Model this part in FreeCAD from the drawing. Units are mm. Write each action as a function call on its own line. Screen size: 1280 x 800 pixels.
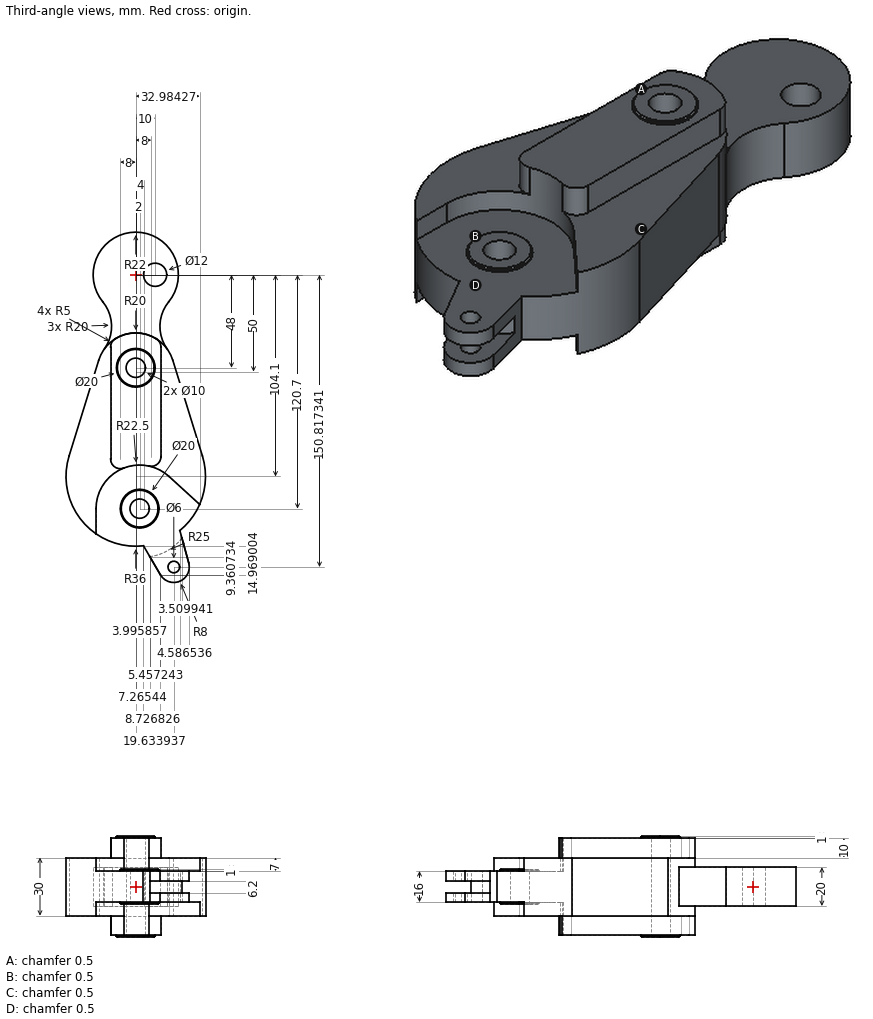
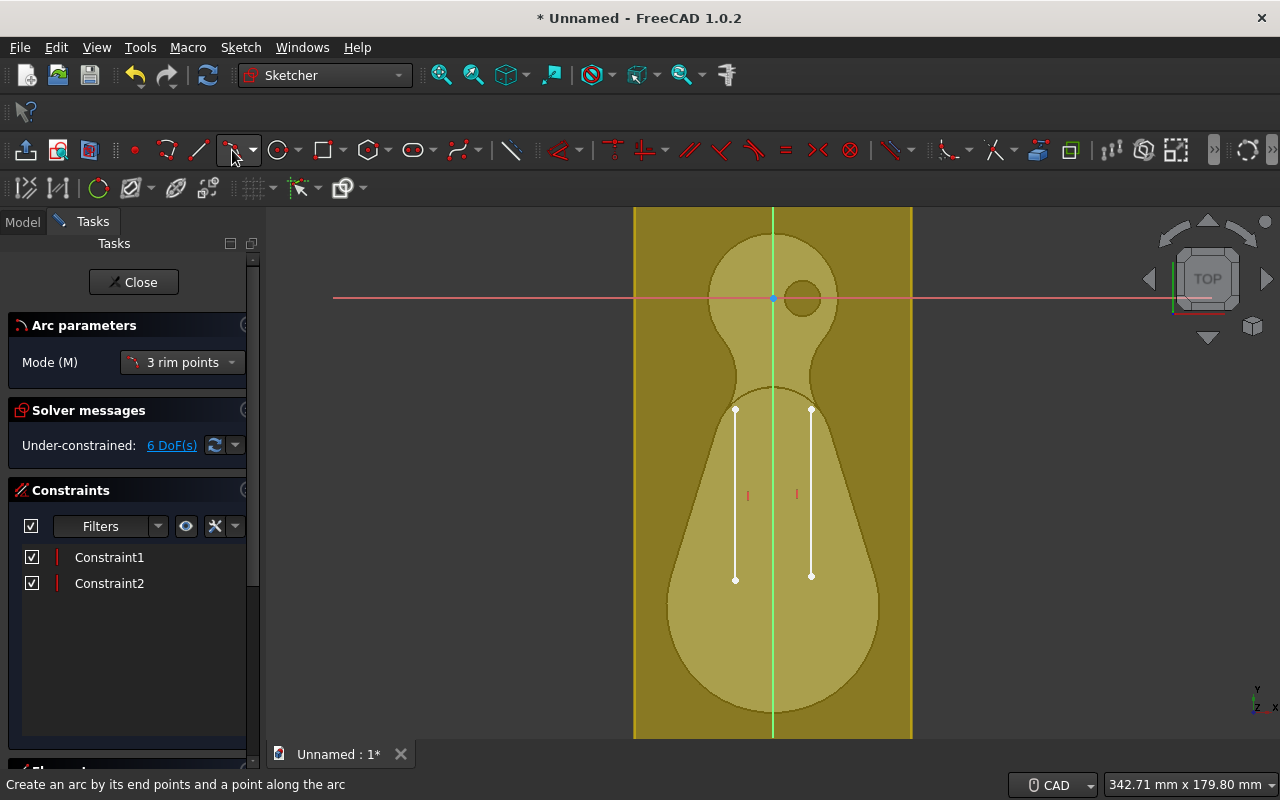
click(735, 581)
click(755, 594)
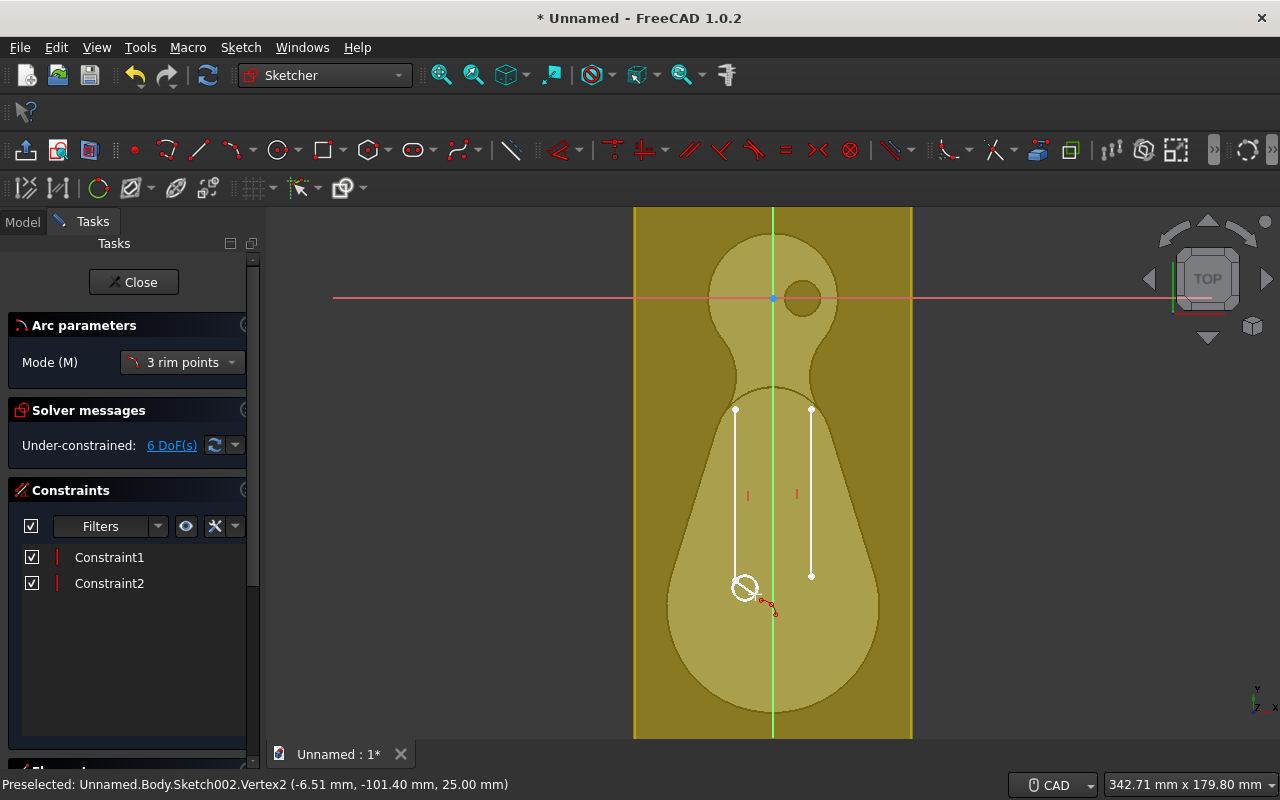
scroll(741, 592, up, 5)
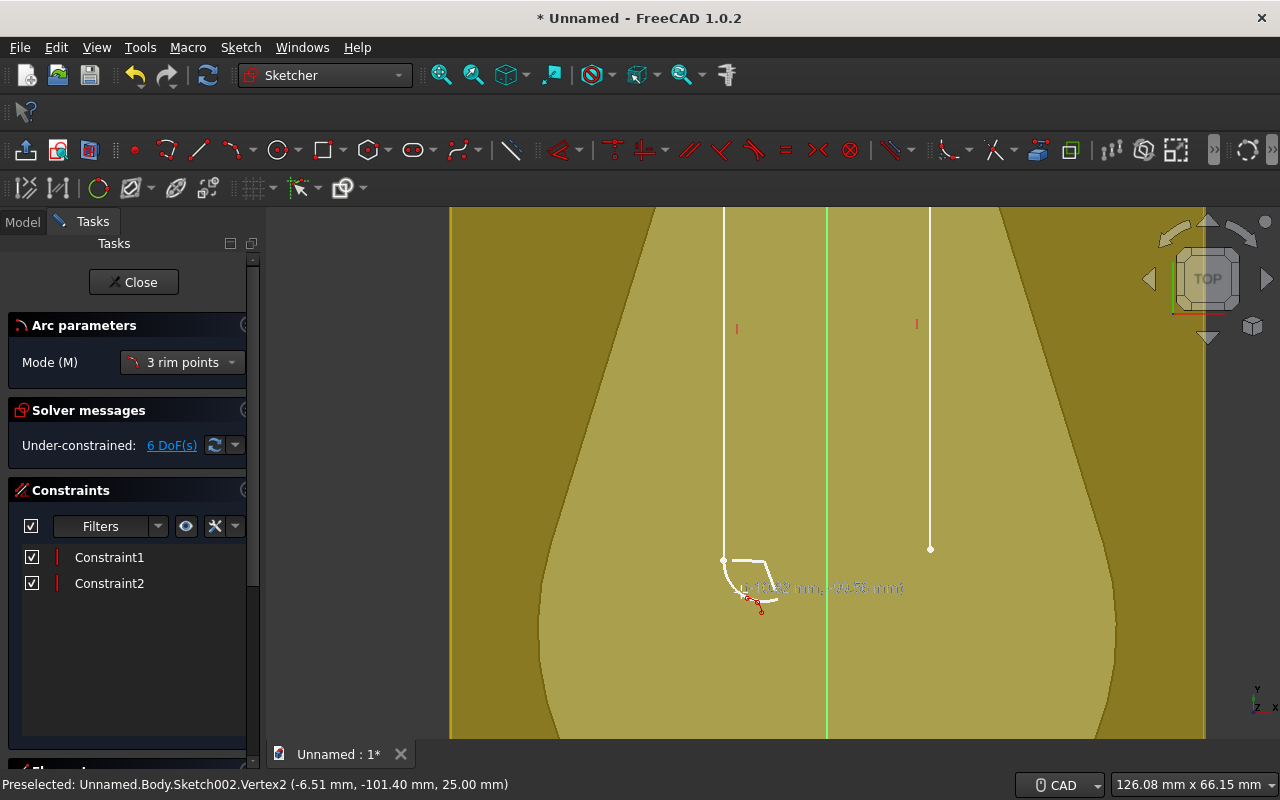
click(740, 591)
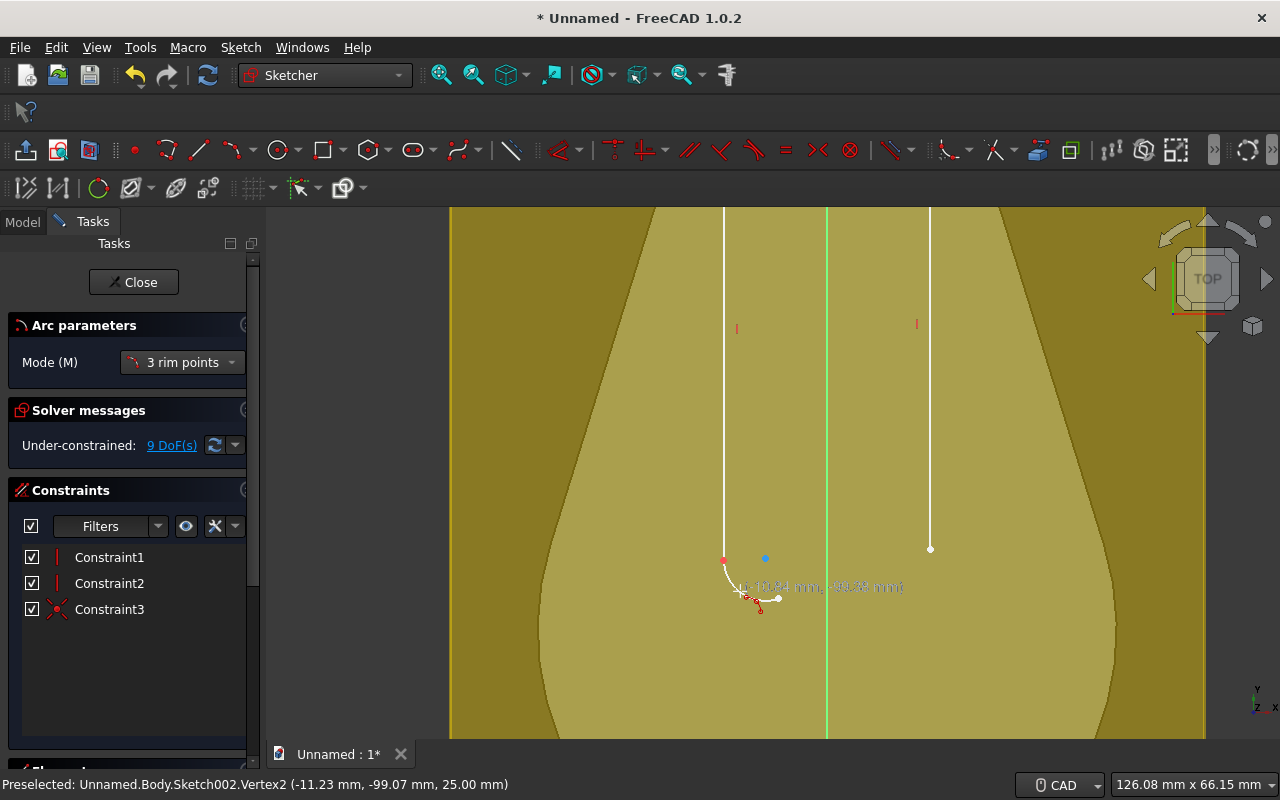
click(778, 599)
click(883, 587)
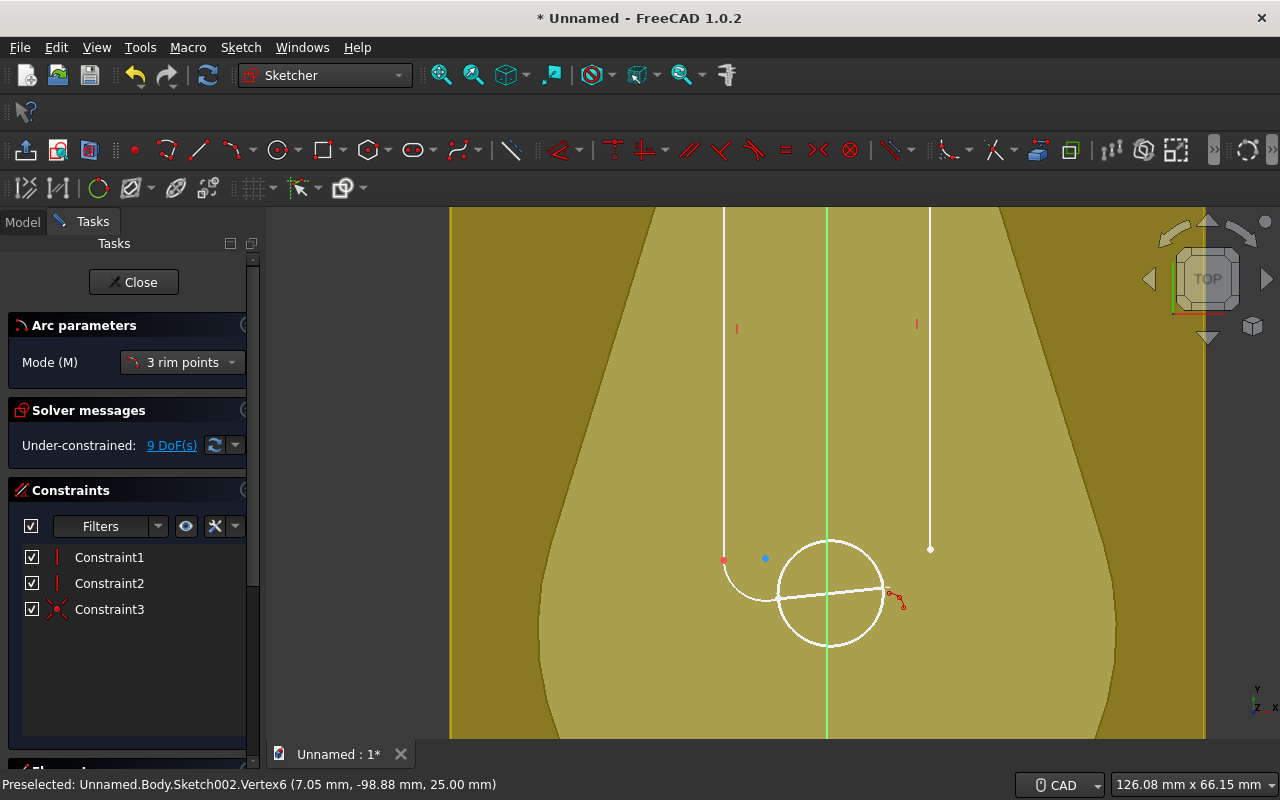
scroll(840, 583, up, 4)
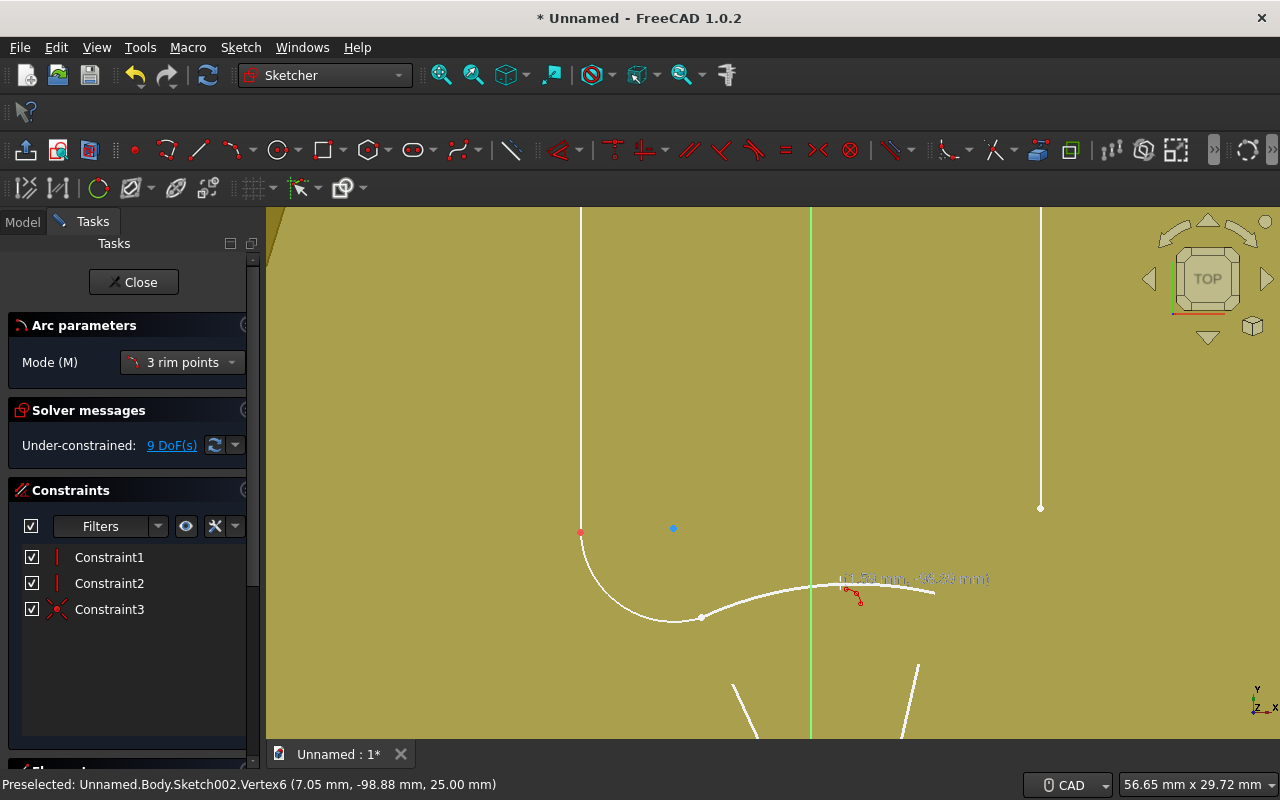
click(840, 581)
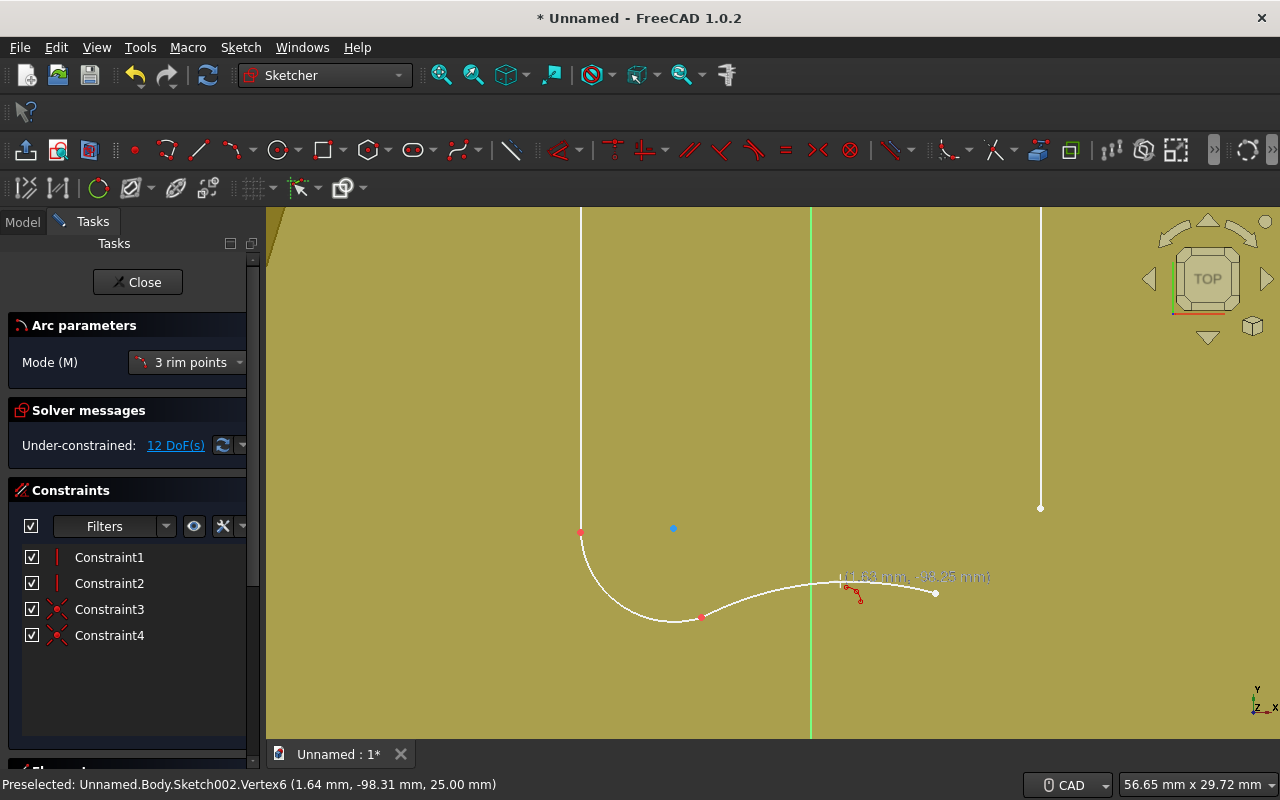
scroll(678, 665, down, 8)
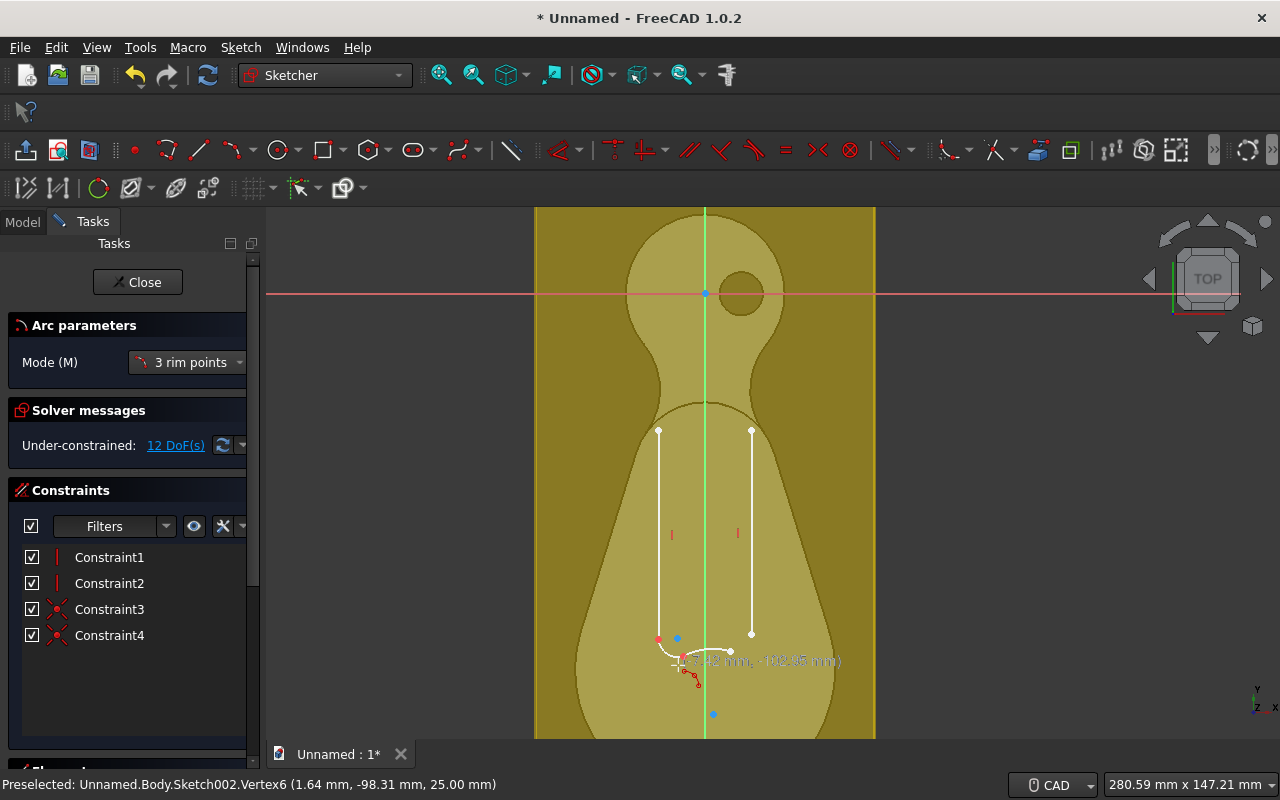
click(730, 651)
click(752, 634)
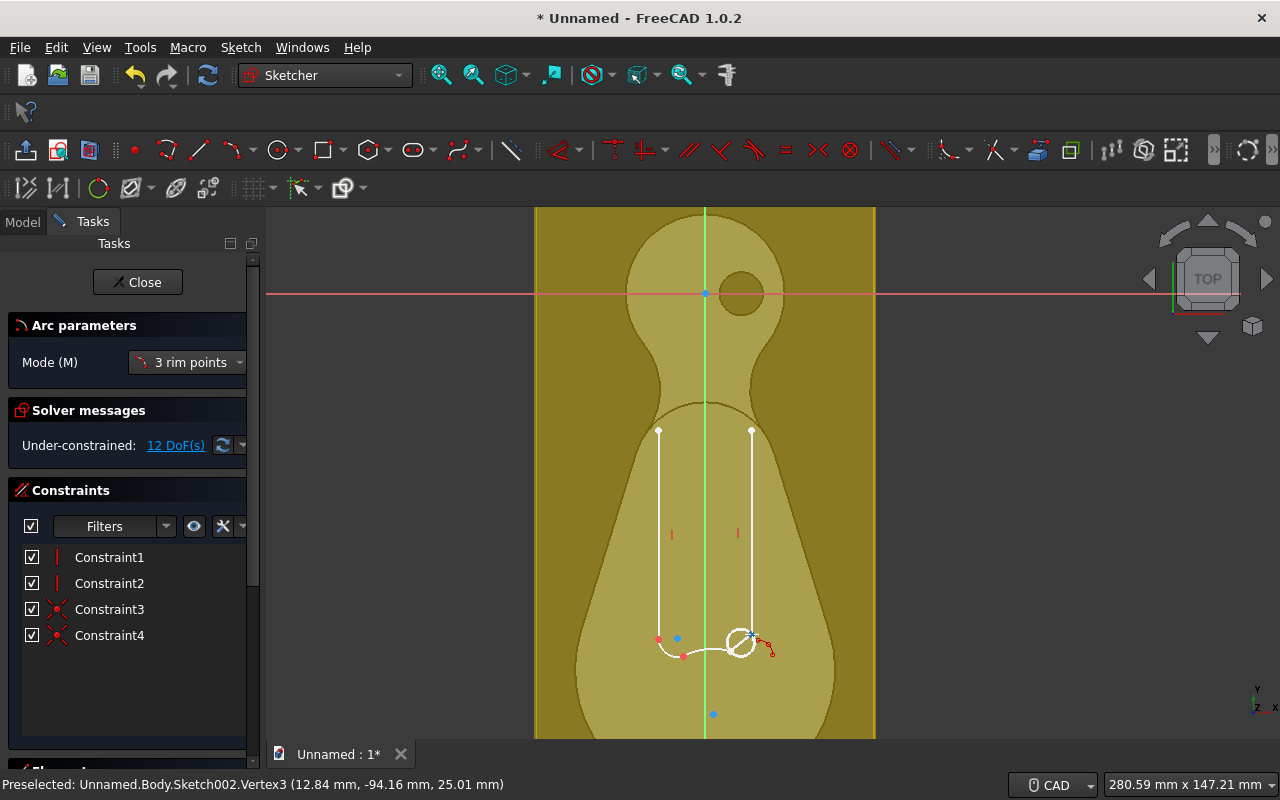
scroll(745, 647, up, 5)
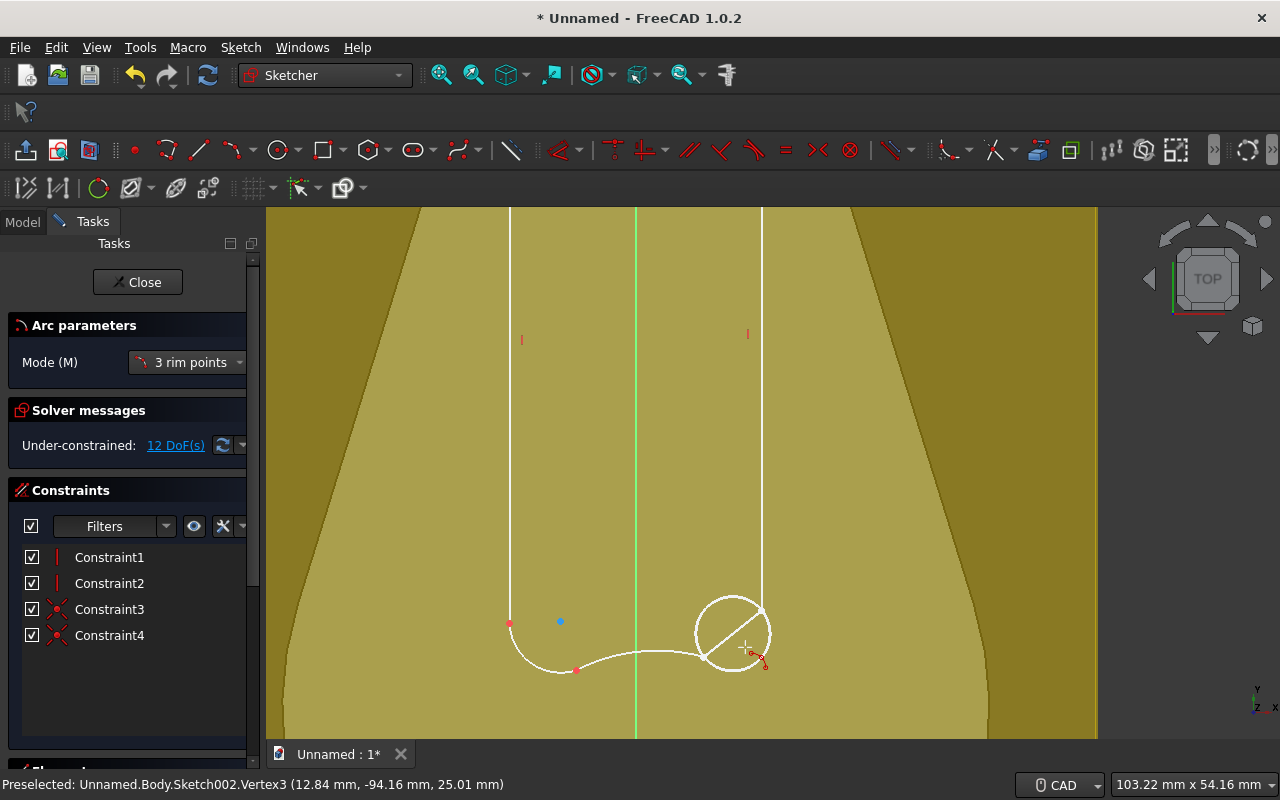
click(745, 646)